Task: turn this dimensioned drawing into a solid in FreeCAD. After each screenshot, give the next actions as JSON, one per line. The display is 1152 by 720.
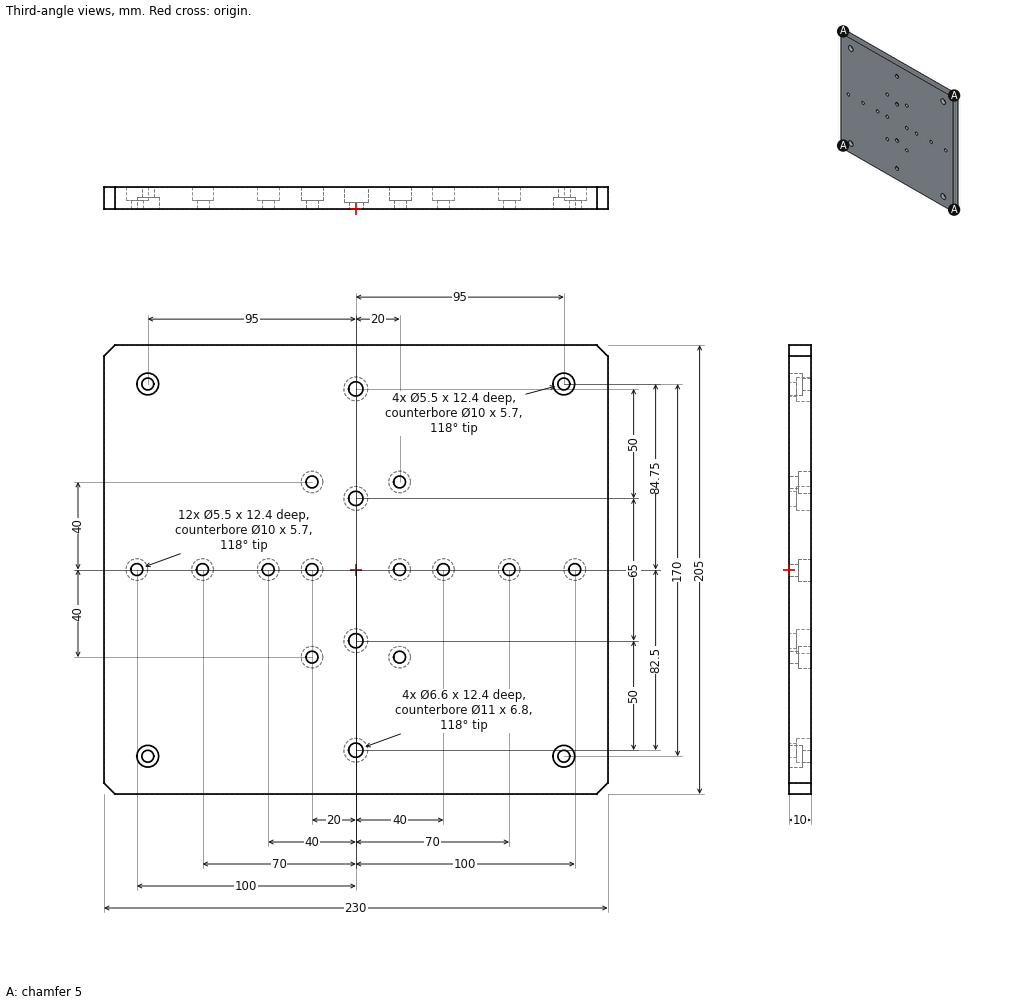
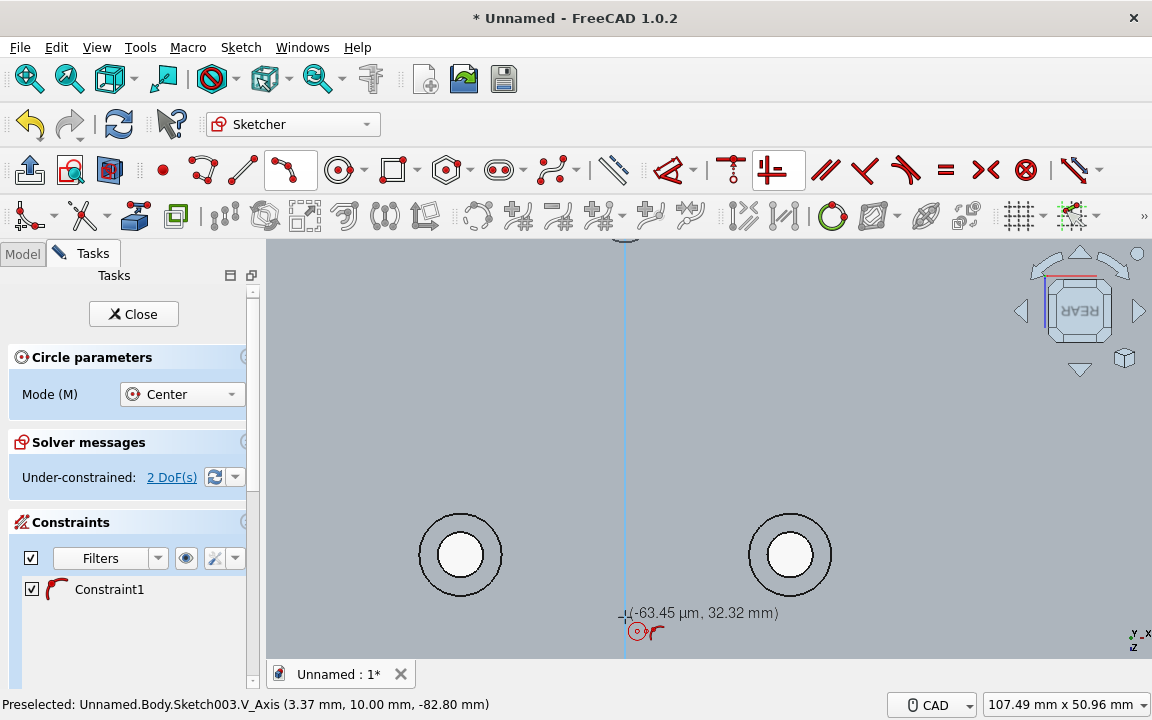
{"action": "scroll", "coordinate": [644, 363], "scroll_direction": "down", "scroll_amount": 9}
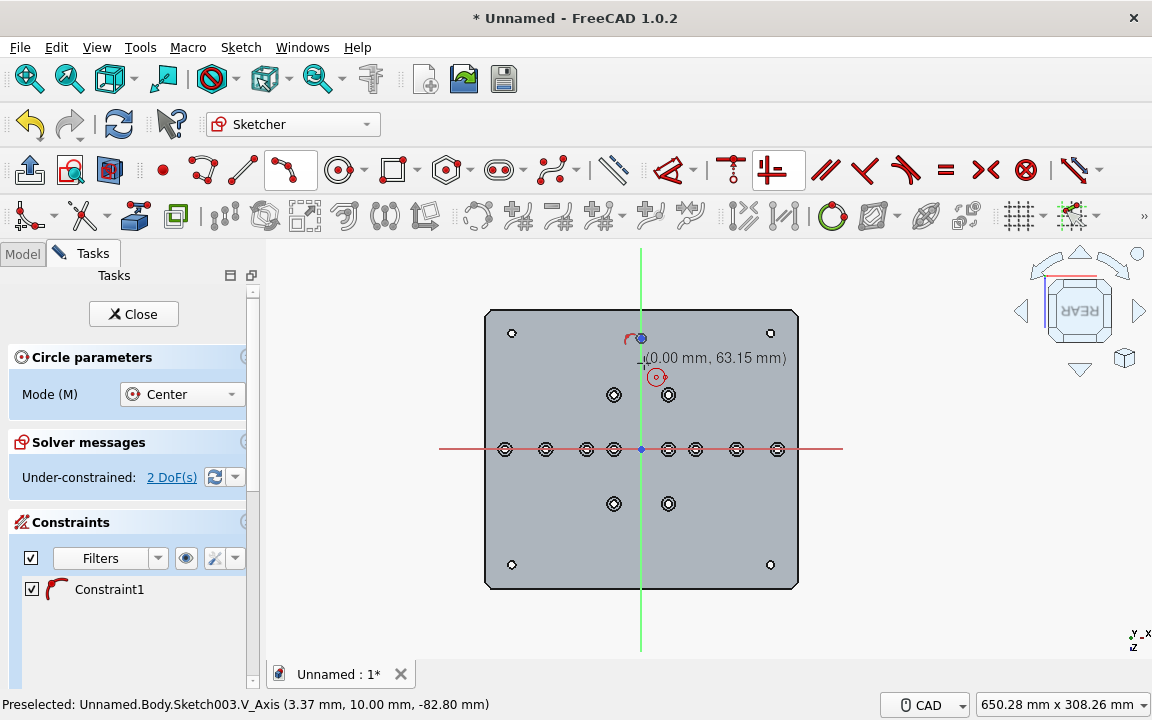
{"action": "left_click", "coordinate": [641, 405]}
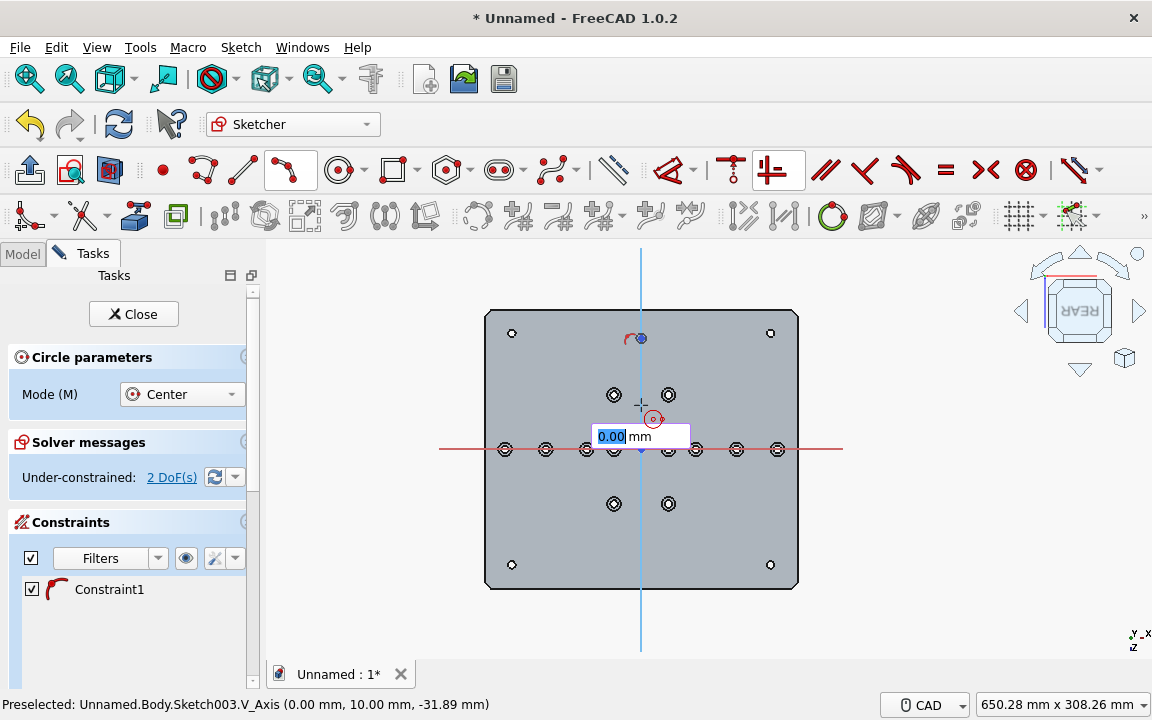
{"action": "scroll", "coordinate": [645, 404], "scroll_direction": "up", "scroll_amount": 7}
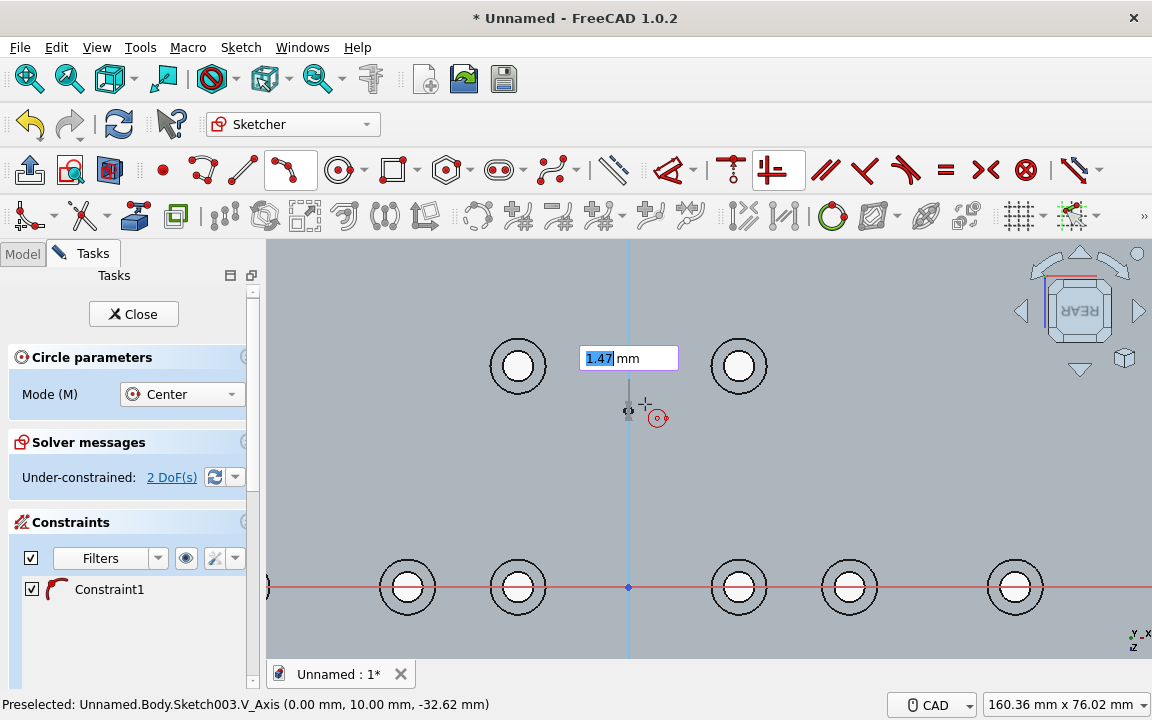
{"action": "left_click", "coordinate": [646, 401]}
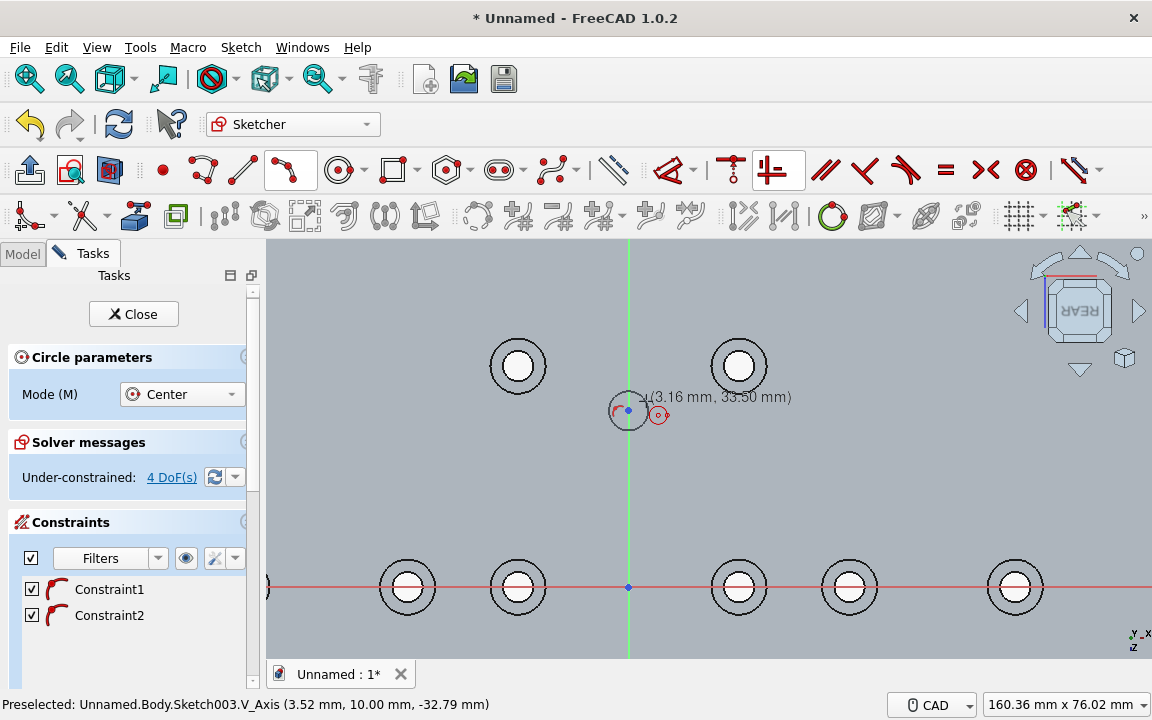
{"action": "scroll", "coordinate": [644, 404], "scroll_direction": "down", "scroll_amount": 7}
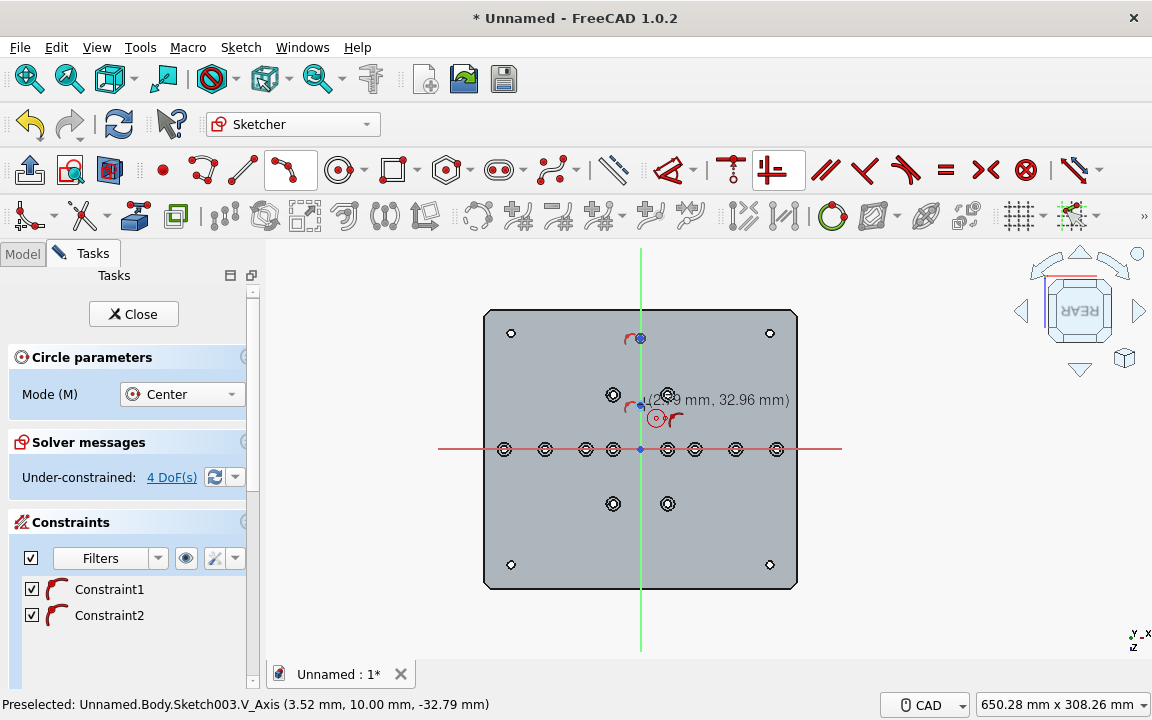
{"action": "scroll", "coordinate": [641, 494], "scroll_direction": "up", "scroll_amount": 9}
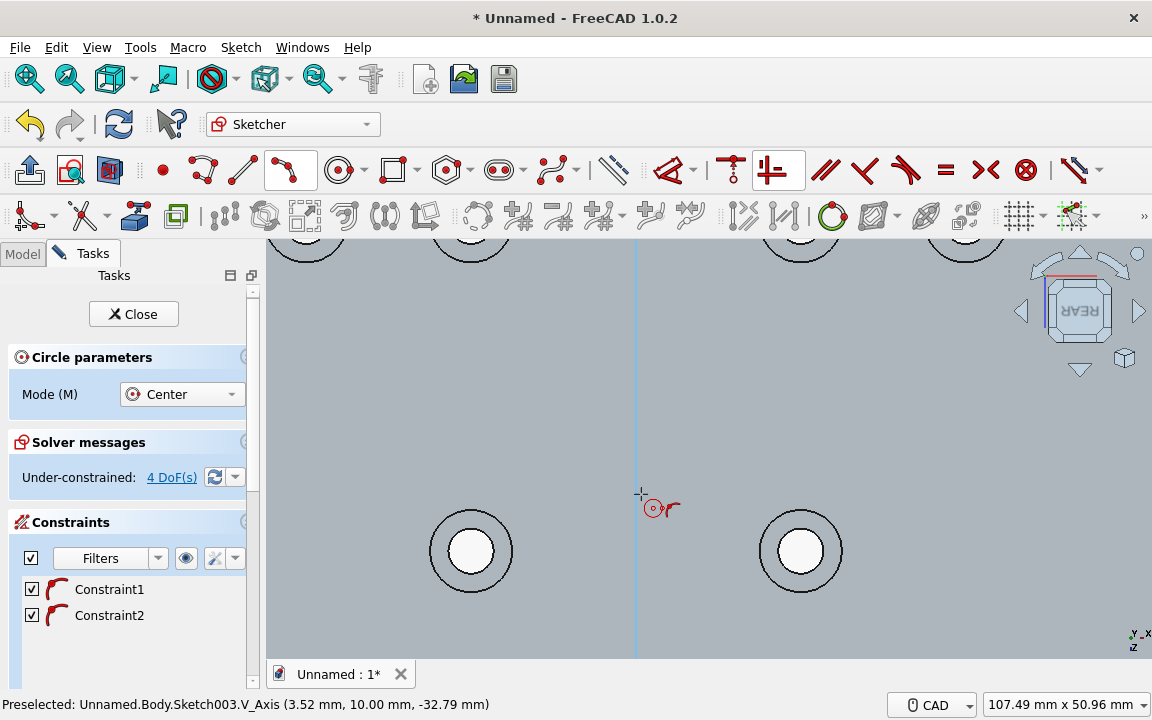
{"action": "scroll", "coordinate": [641, 494], "scroll_direction": "down", "scroll_amount": 9}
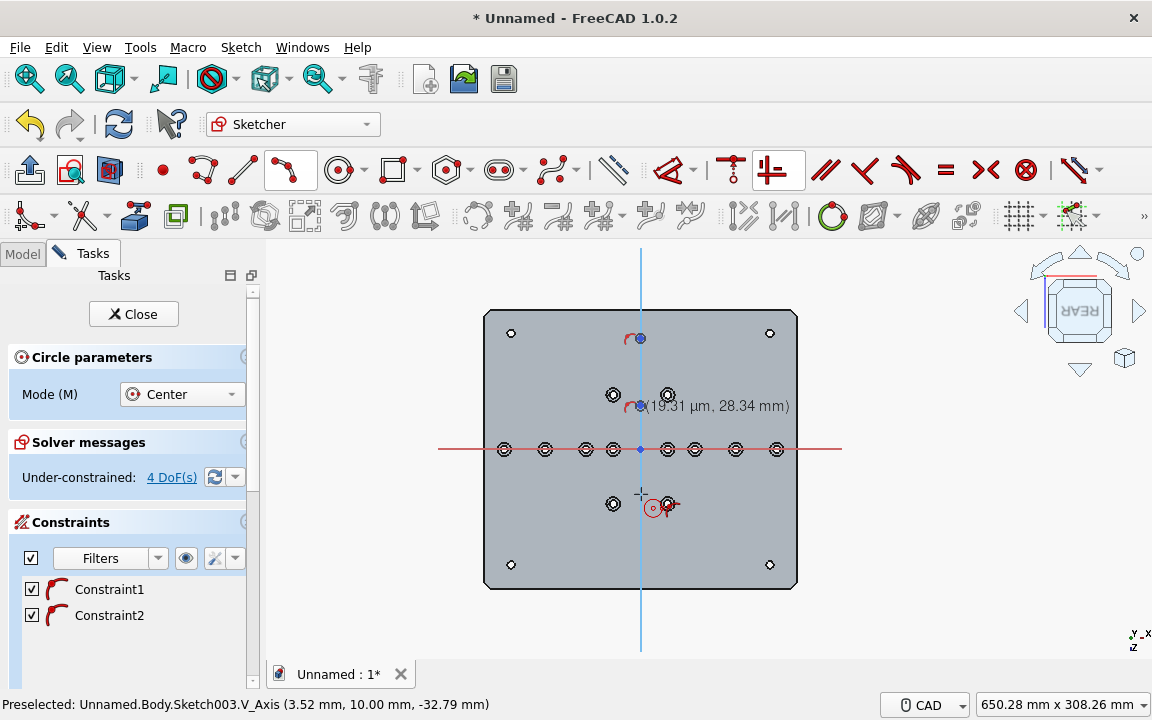
{"action": "left_click", "coordinate": [641, 494]}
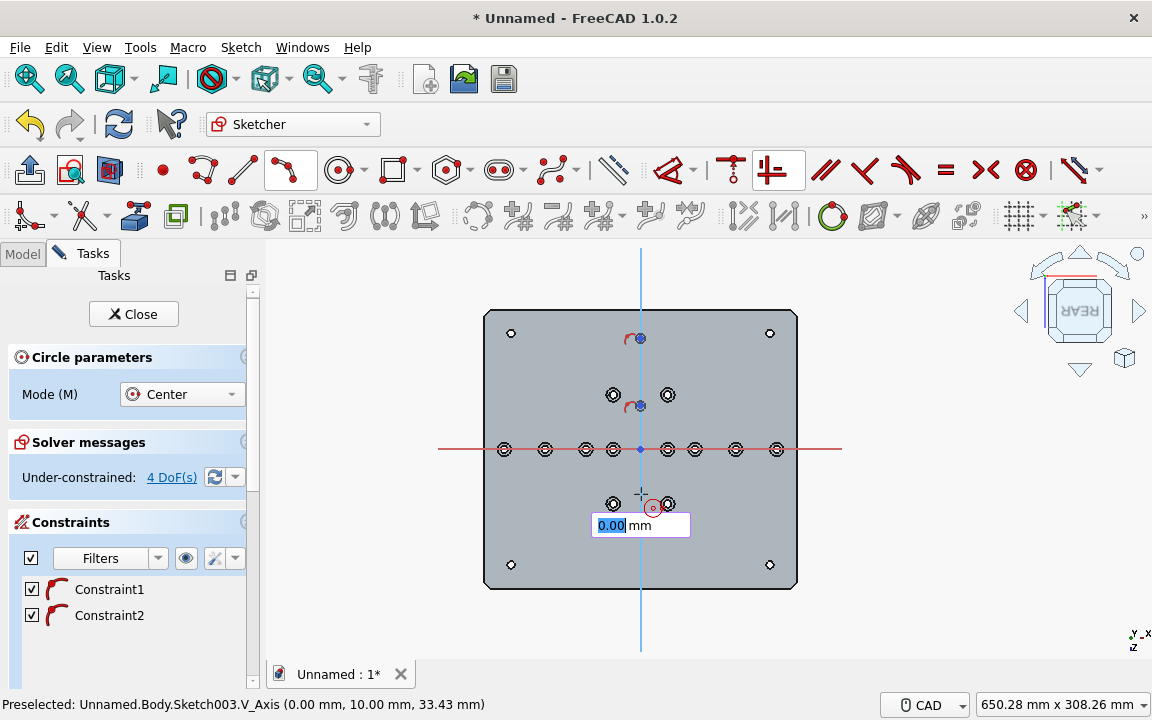
{"action": "scroll", "coordinate": [645, 492], "scroll_direction": "up", "scroll_amount": 7}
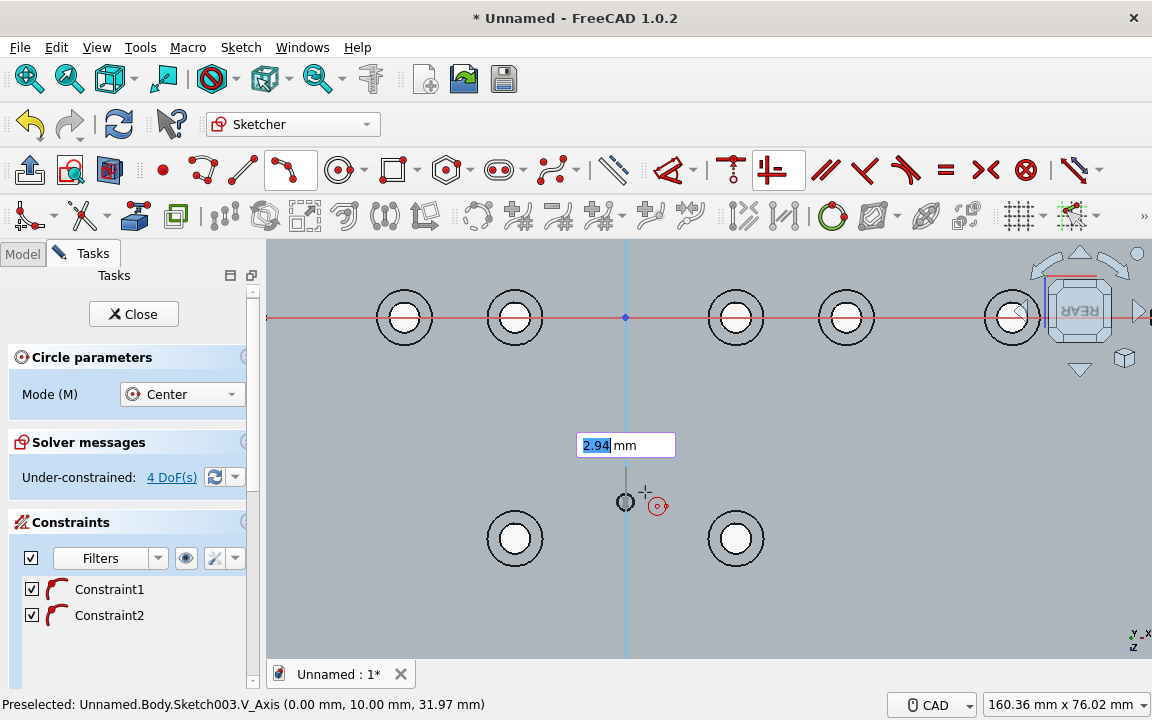
{"action": "left_click", "coordinate": [643, 491]}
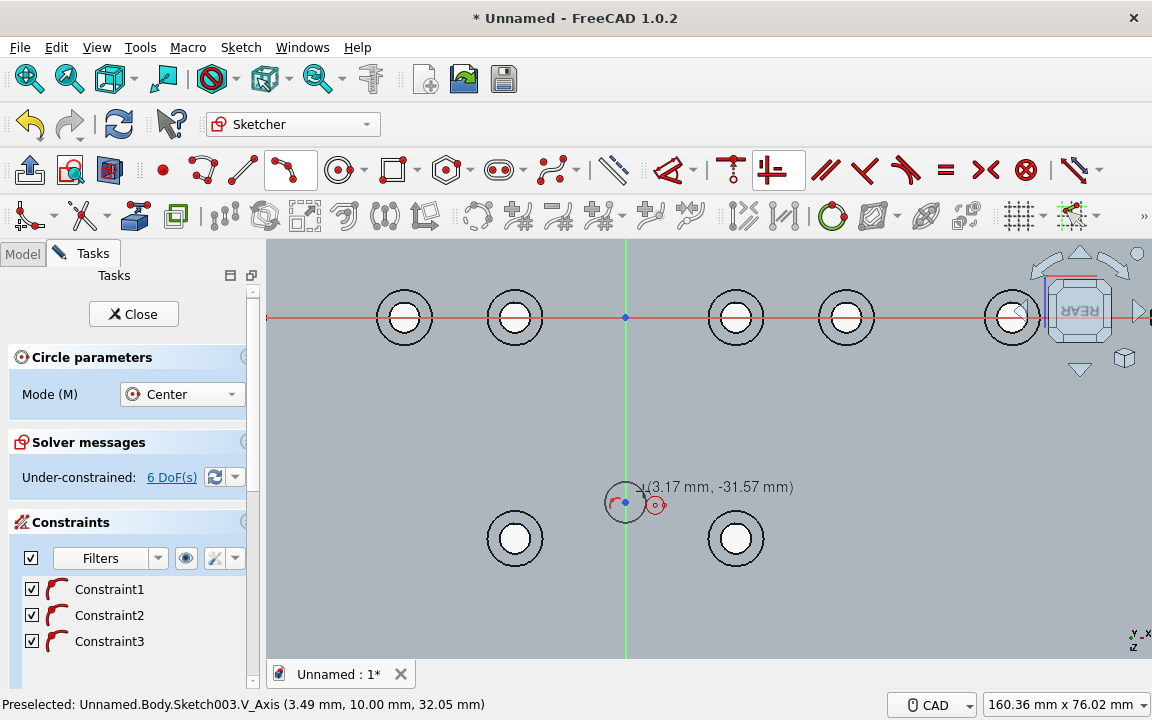
{"action": "scroll", "coordinate": [645, 492], "scroll_direction": "down", "scroll_amount": 7}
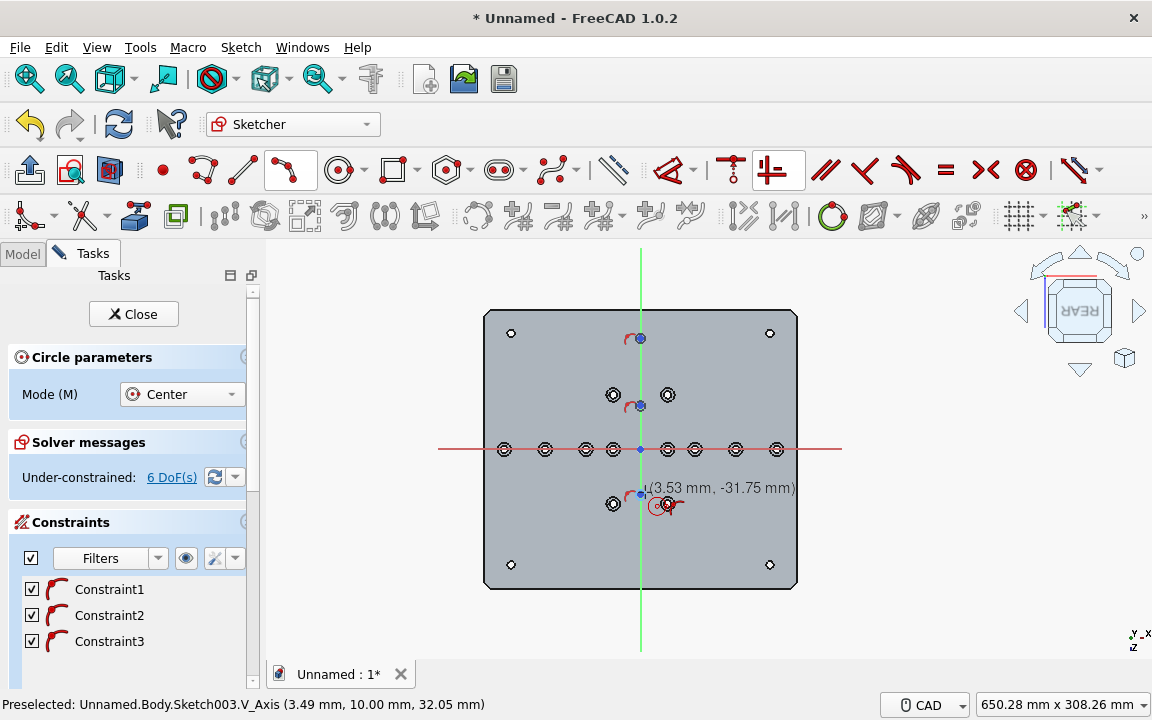
{"action": "scroll", "coordinate": [641, 562], "scroll_direction": "up", "scroll_amount": 9}